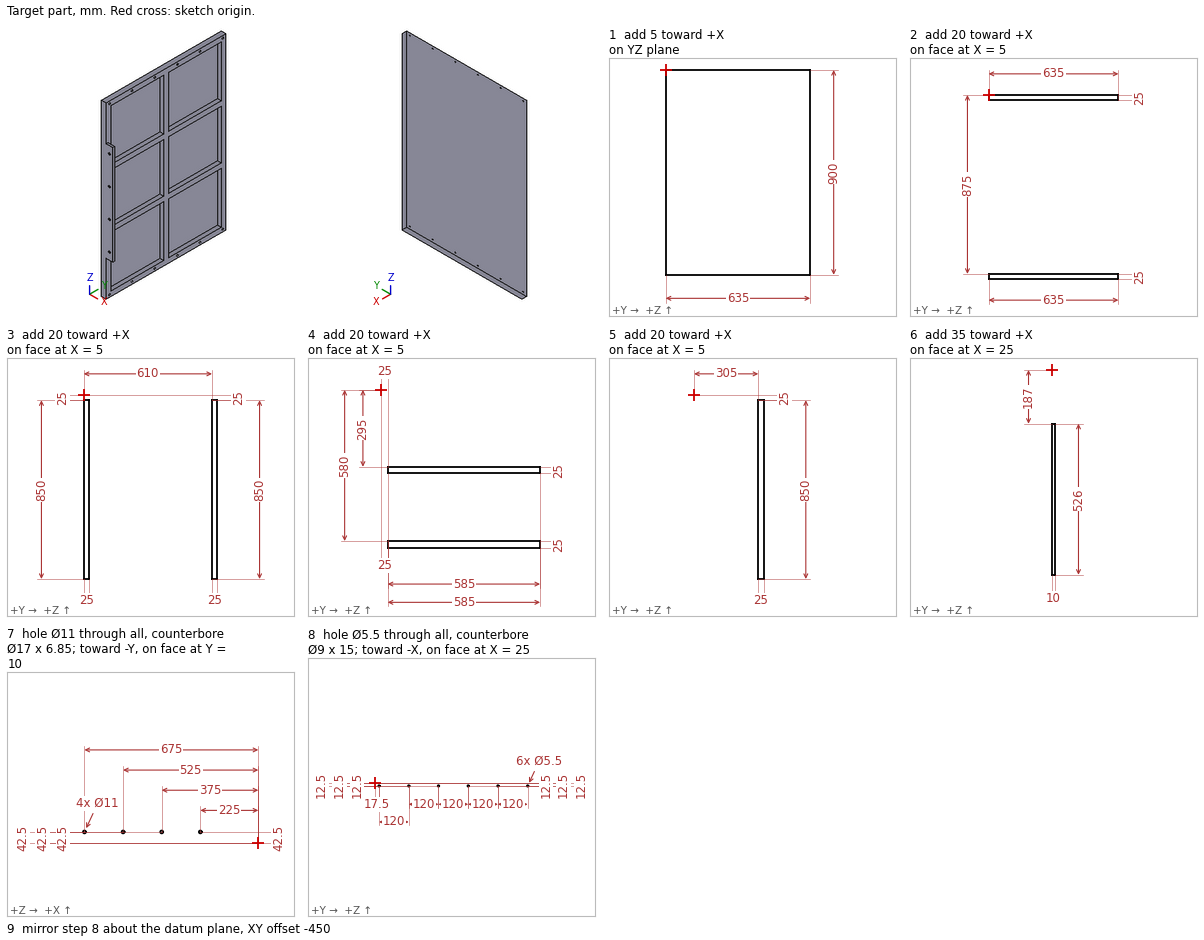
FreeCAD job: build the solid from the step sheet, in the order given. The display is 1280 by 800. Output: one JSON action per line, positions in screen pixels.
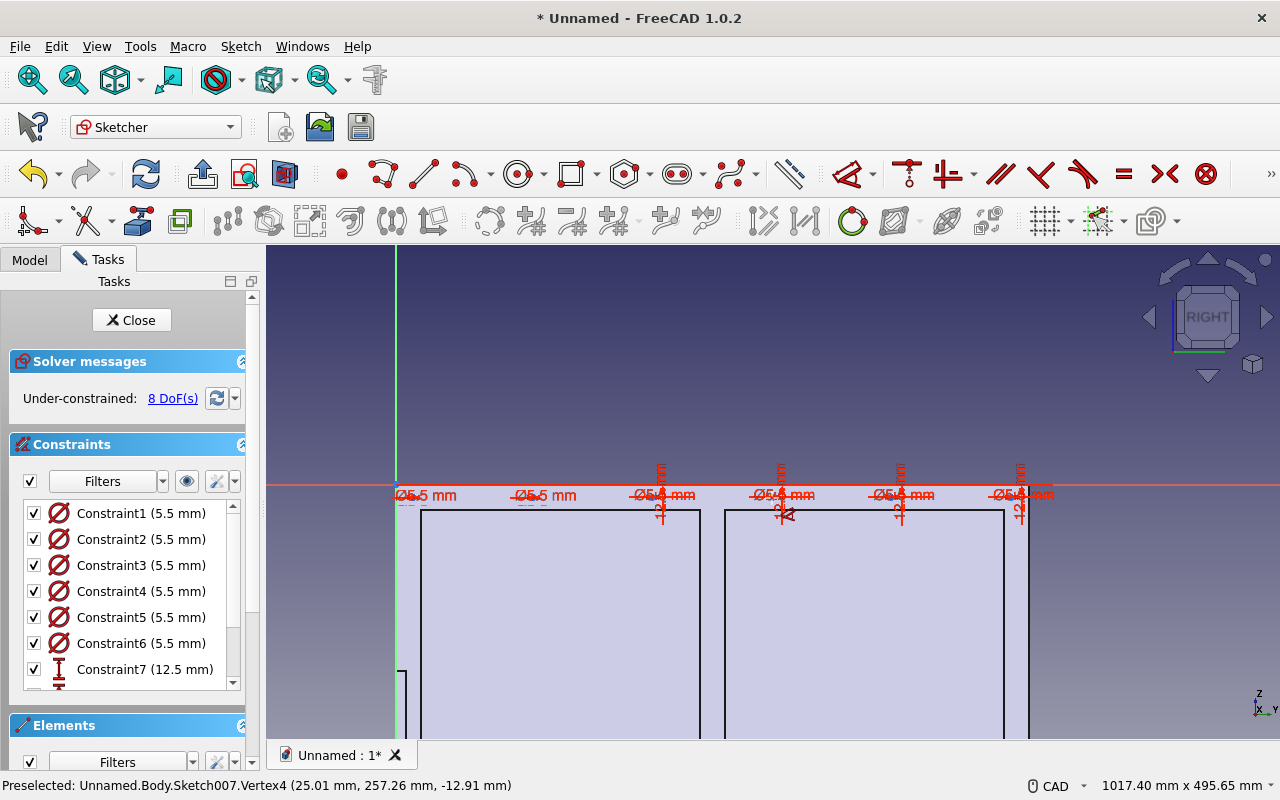
{"action": "scroll", "coordinate": [533, 498], "scroll_direction": "up", "scroll_amount": 6}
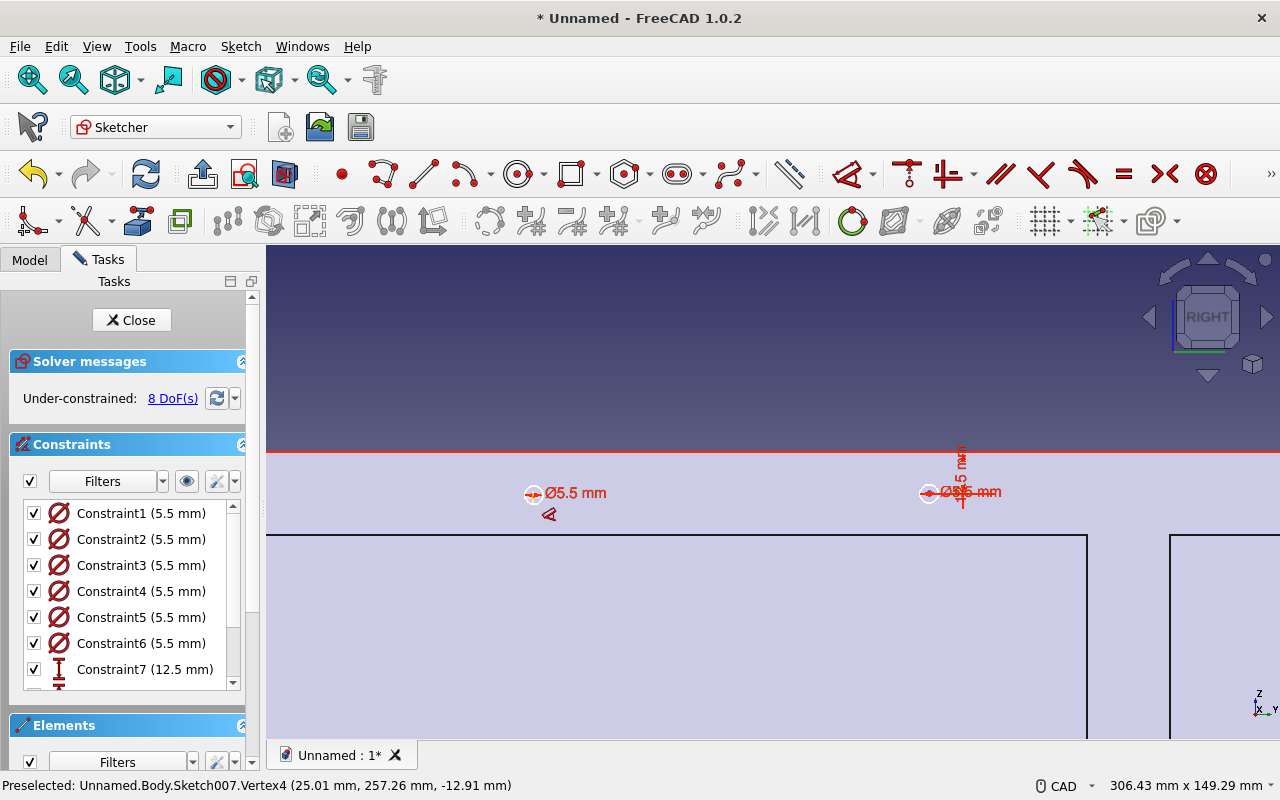
{"action": "left_click", "coordinate": [534, 495]}
{"action": "left_click", "coordinate": [568, 474]}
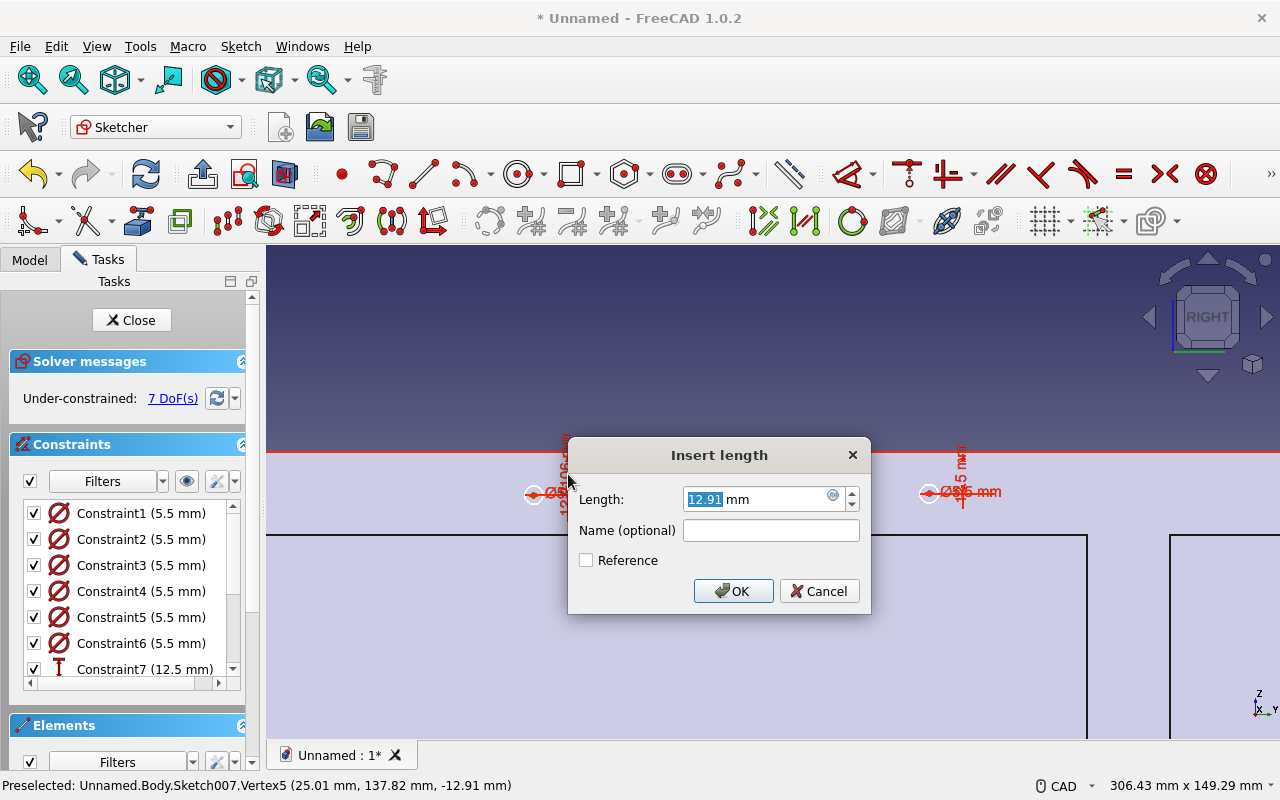
{"action": "type", "text": "12.5"}
{"action": "key", "text": "Return"}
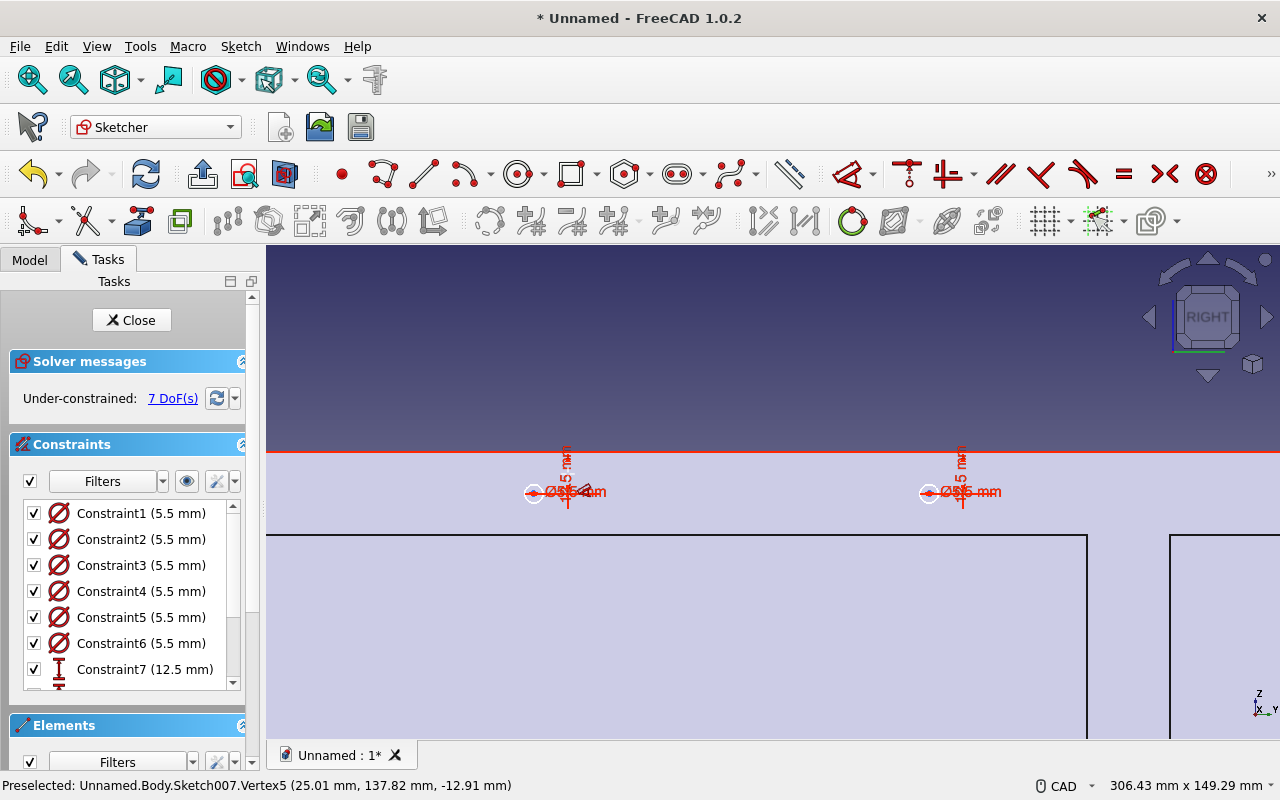
{"action": "scroll", "coordinate": [532, 498], "scroll_direction": "down", "scroll_amount": 6}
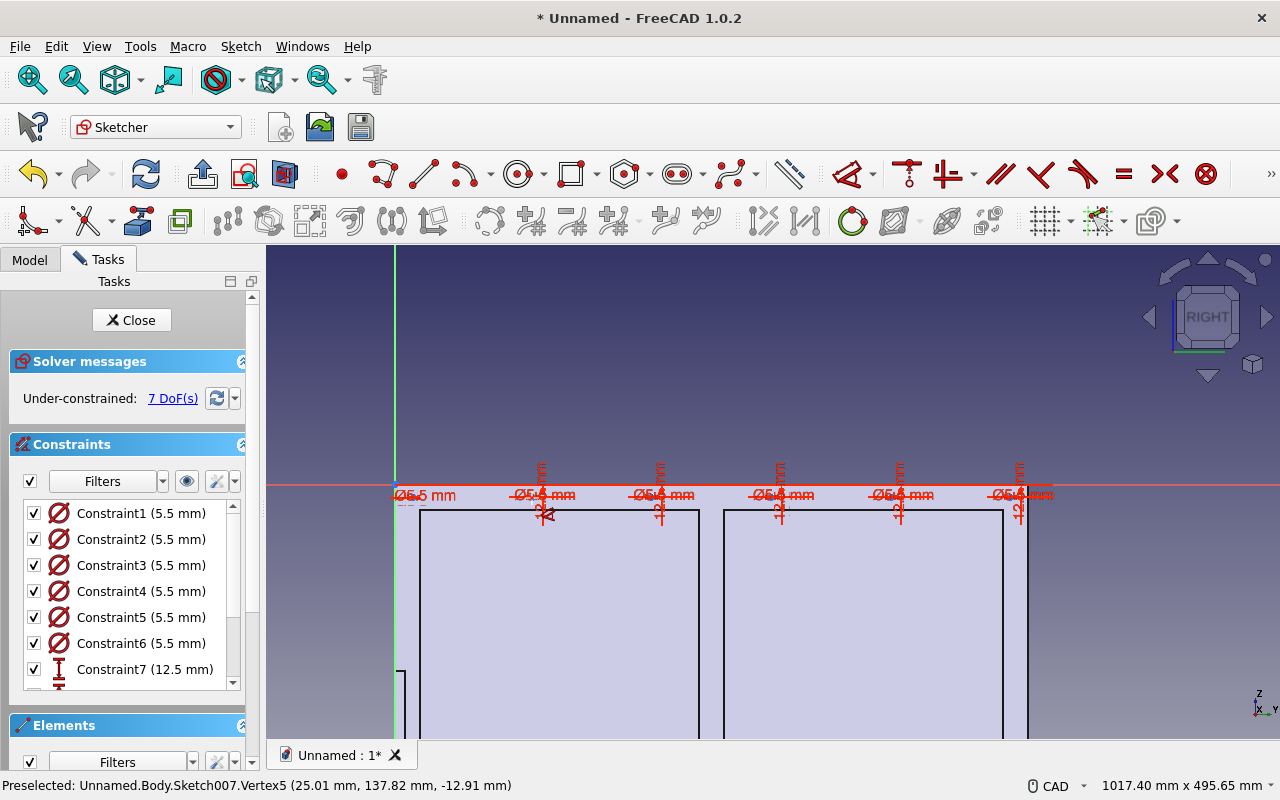
{"action": "scroll", "coordinate": [413, 498], "scroll_direction": "up", "scroll_amount": 5}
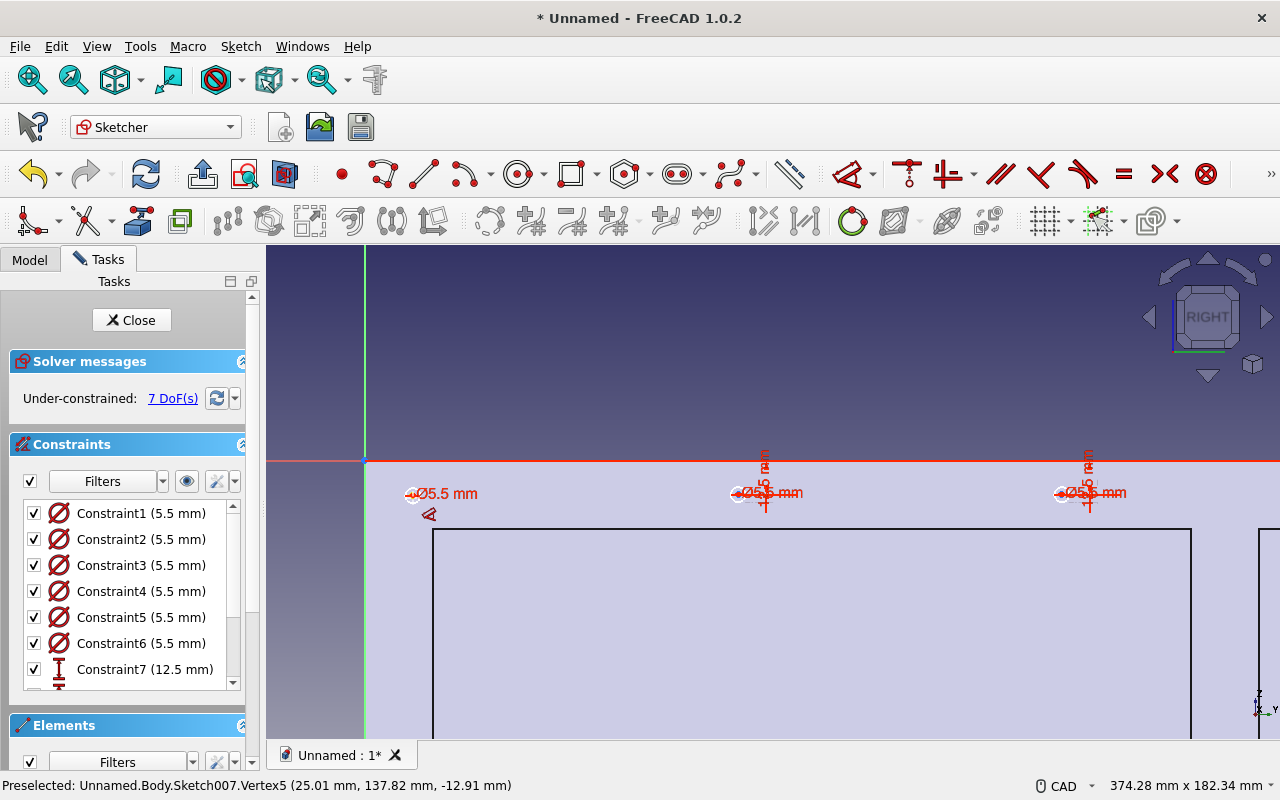
{"action": "left_click", "coordinate": [413, 496]}
{"action": "left_click", "coordinate": [389, 427]}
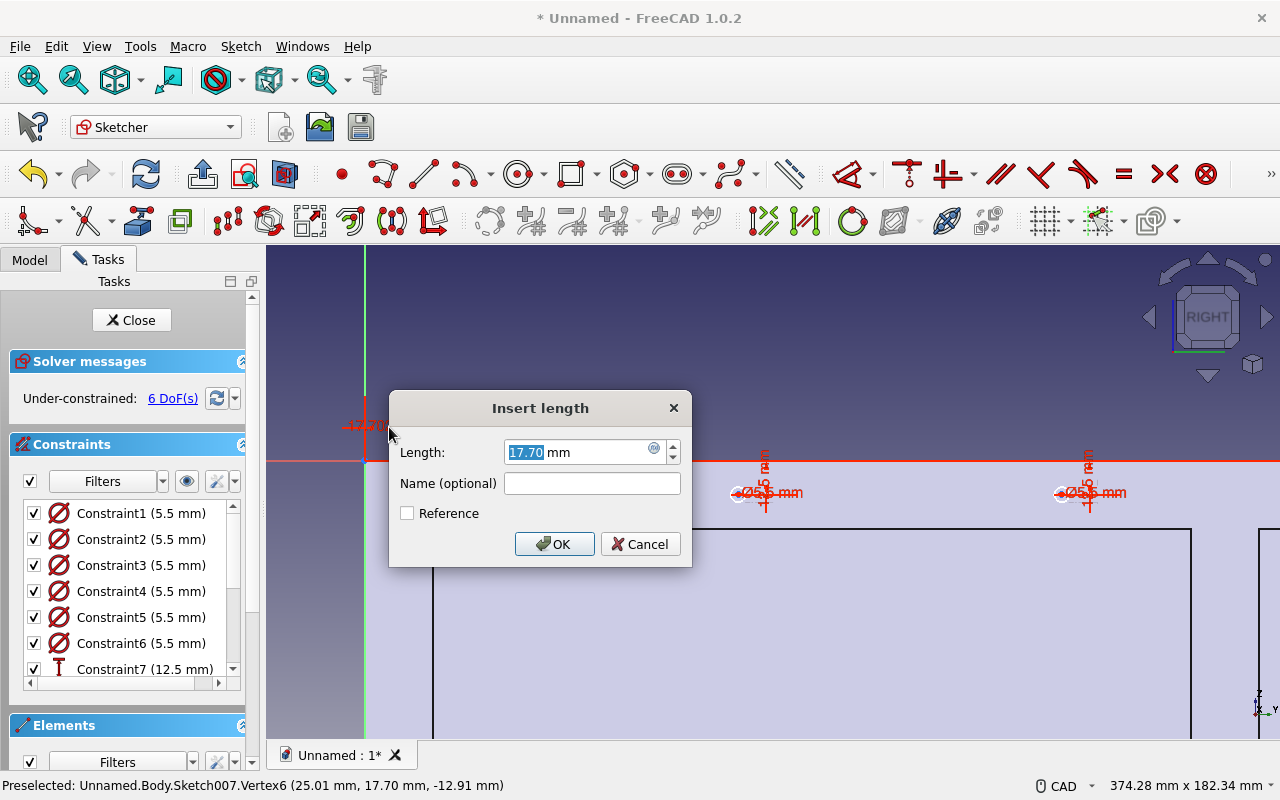
{"action": "type", "text": "17.5"}
{"action": "key", "text": "Return"}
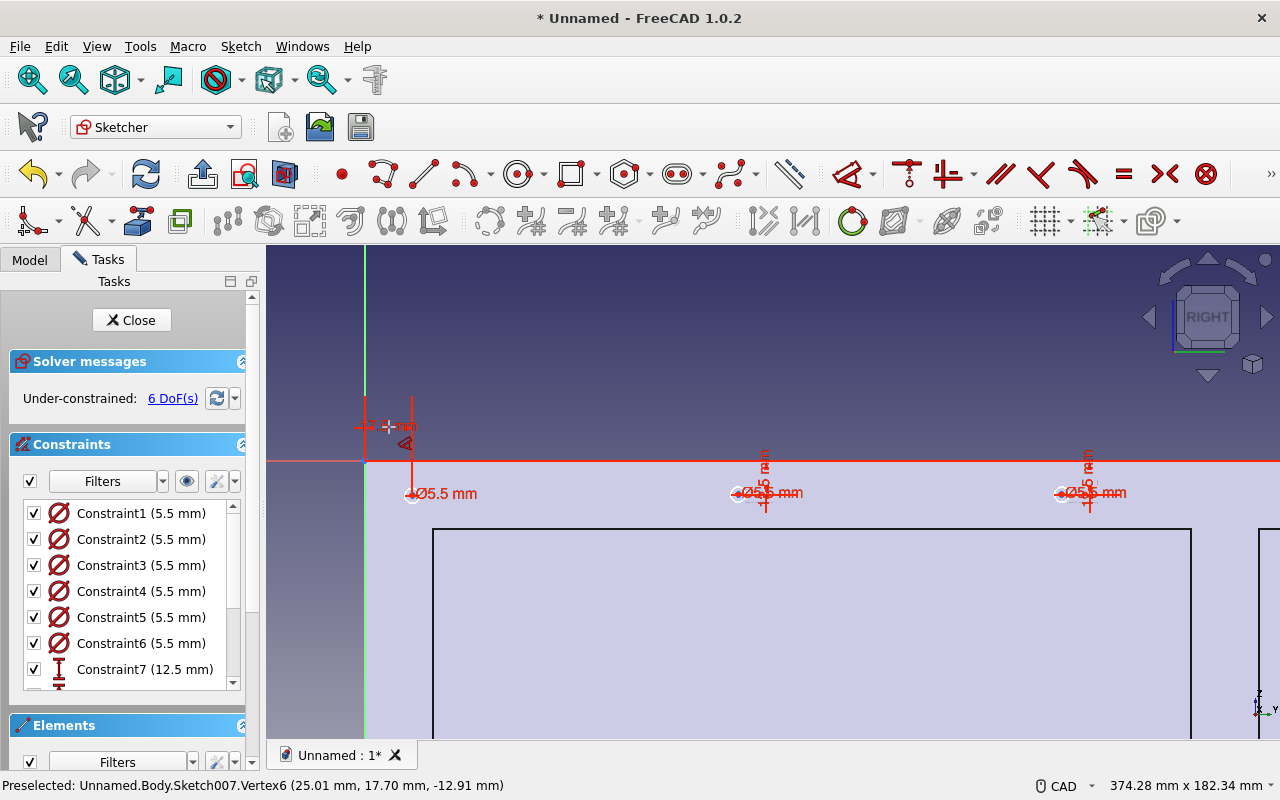
{"action": "left_click", "coordinate": [412, 496]}
{"action": "left_click", "coordinate": [331, 478]}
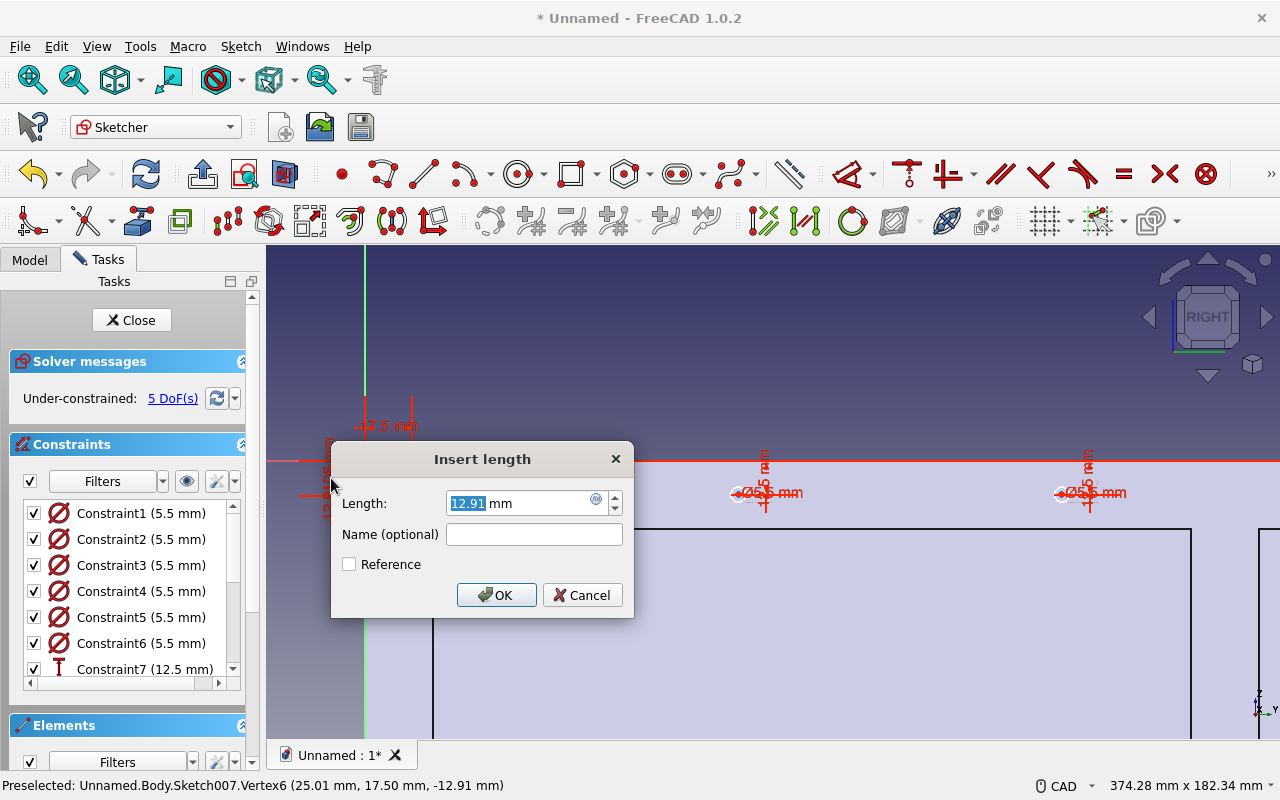
{"action": "type", "text": "12.5"}
{"action": "key", "text": "Return"}